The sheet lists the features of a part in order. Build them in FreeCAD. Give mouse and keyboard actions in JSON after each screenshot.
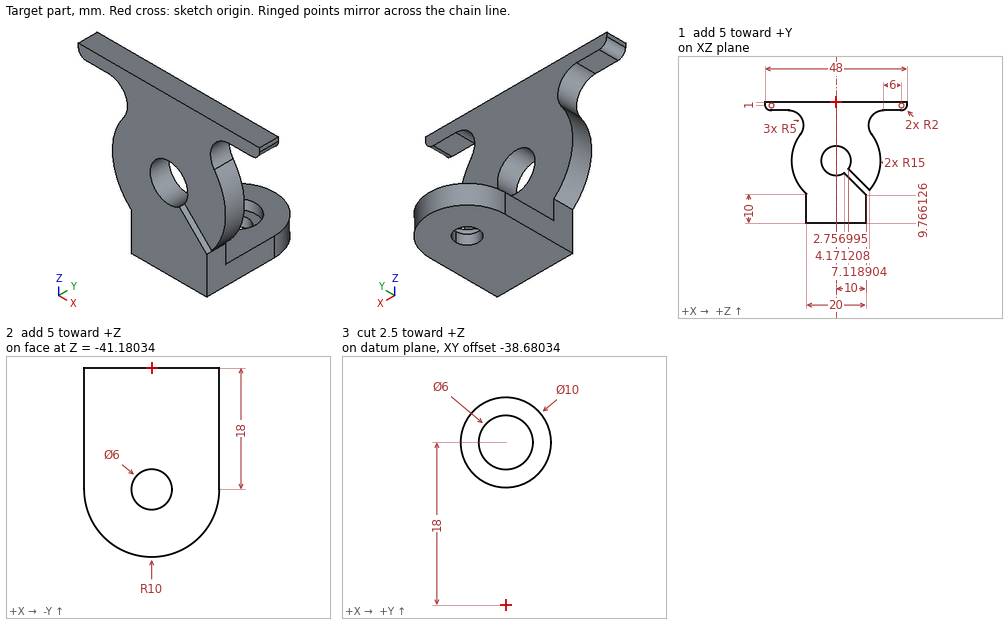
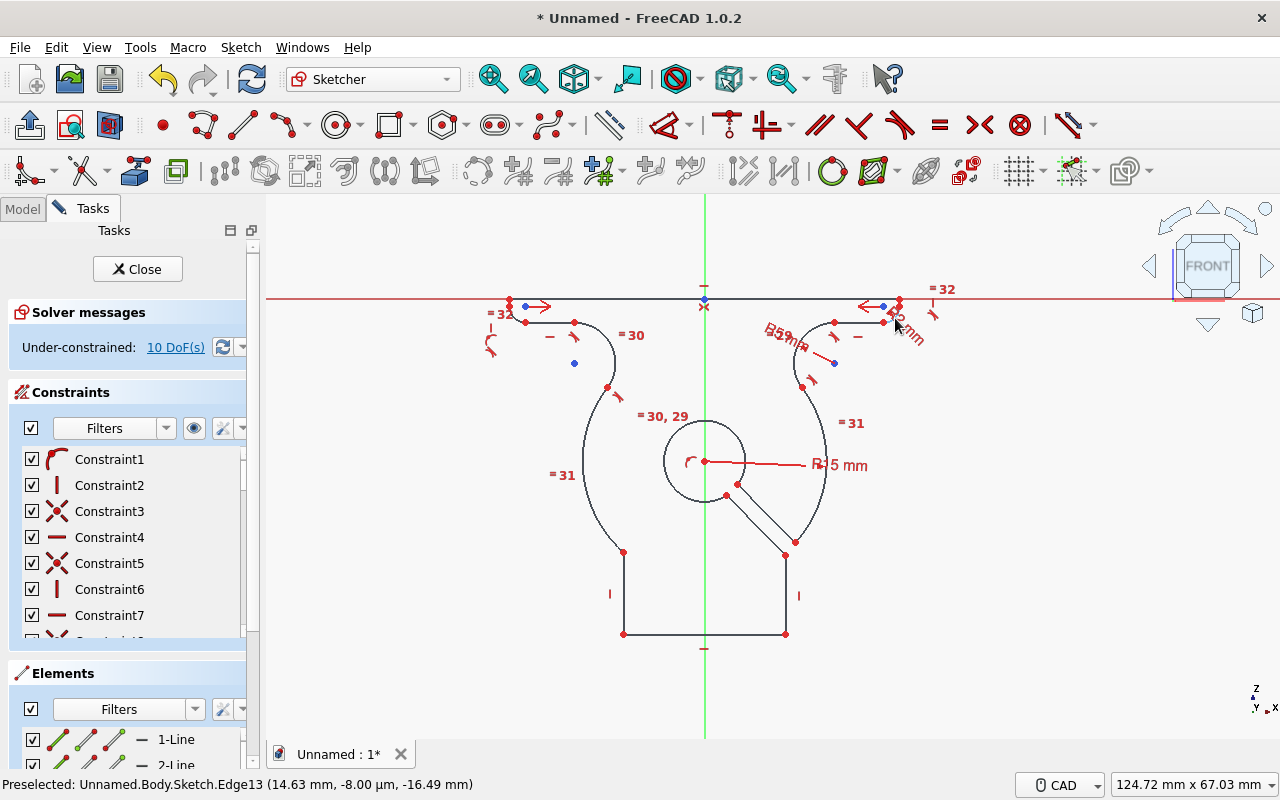
{"action": "scroll", "coordinate": [510, 303], "scroll_direction": "up", "scroll_amount": 8}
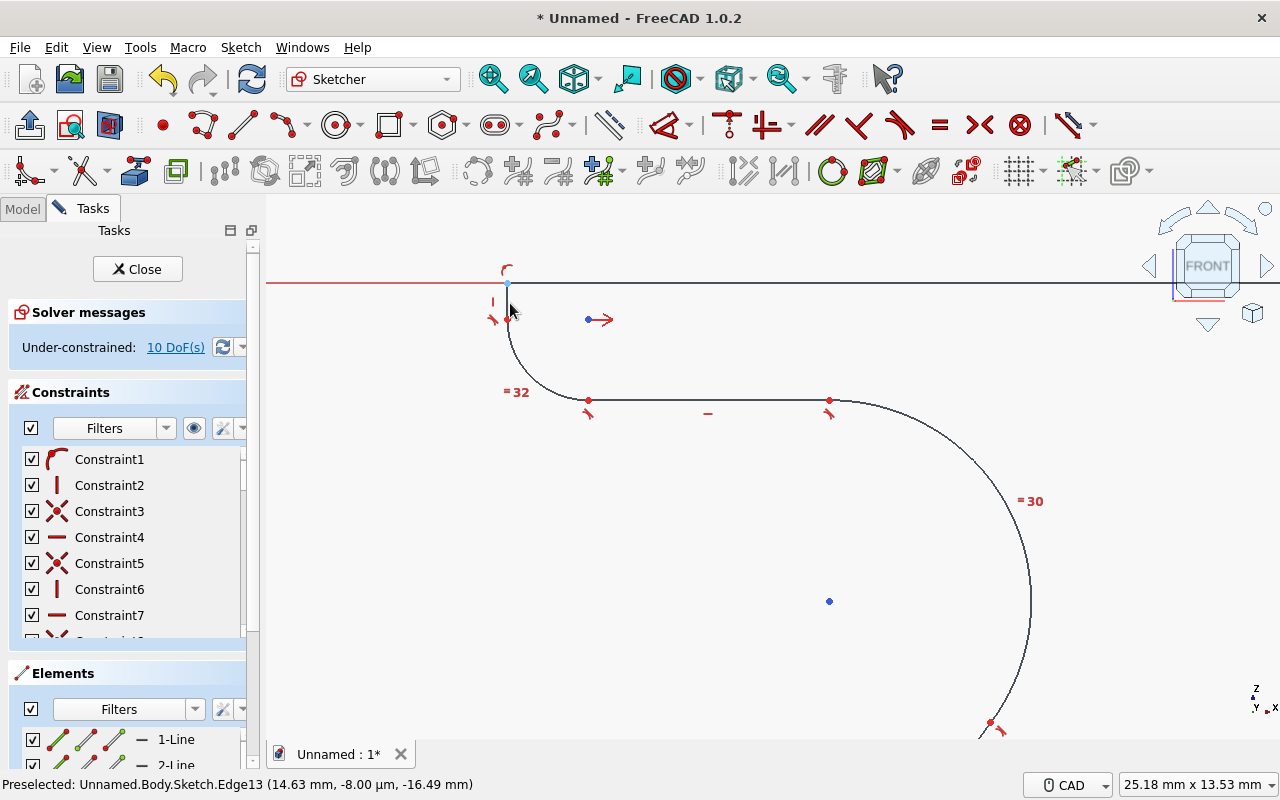
{"action": "left_click", "coordinate": [507, 301]}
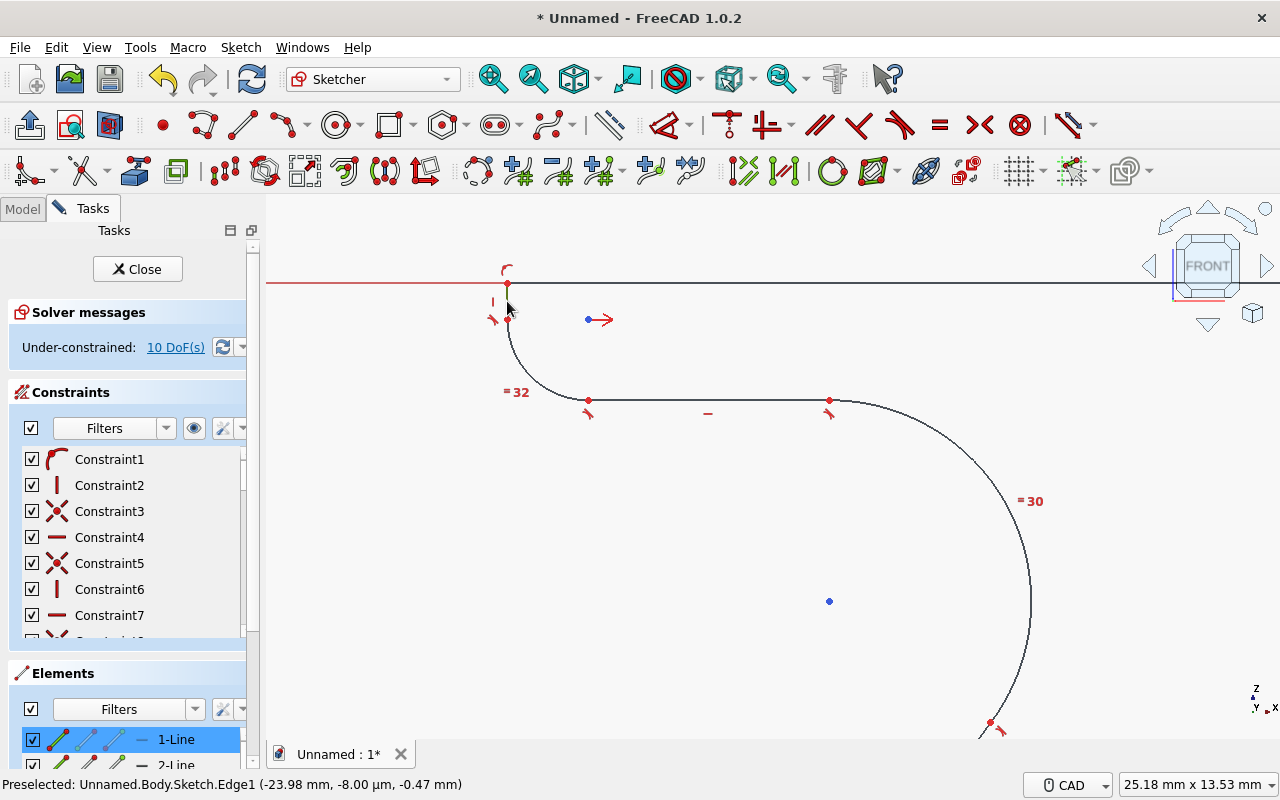
{"action": "left_click", "coordinate": [692, 126]}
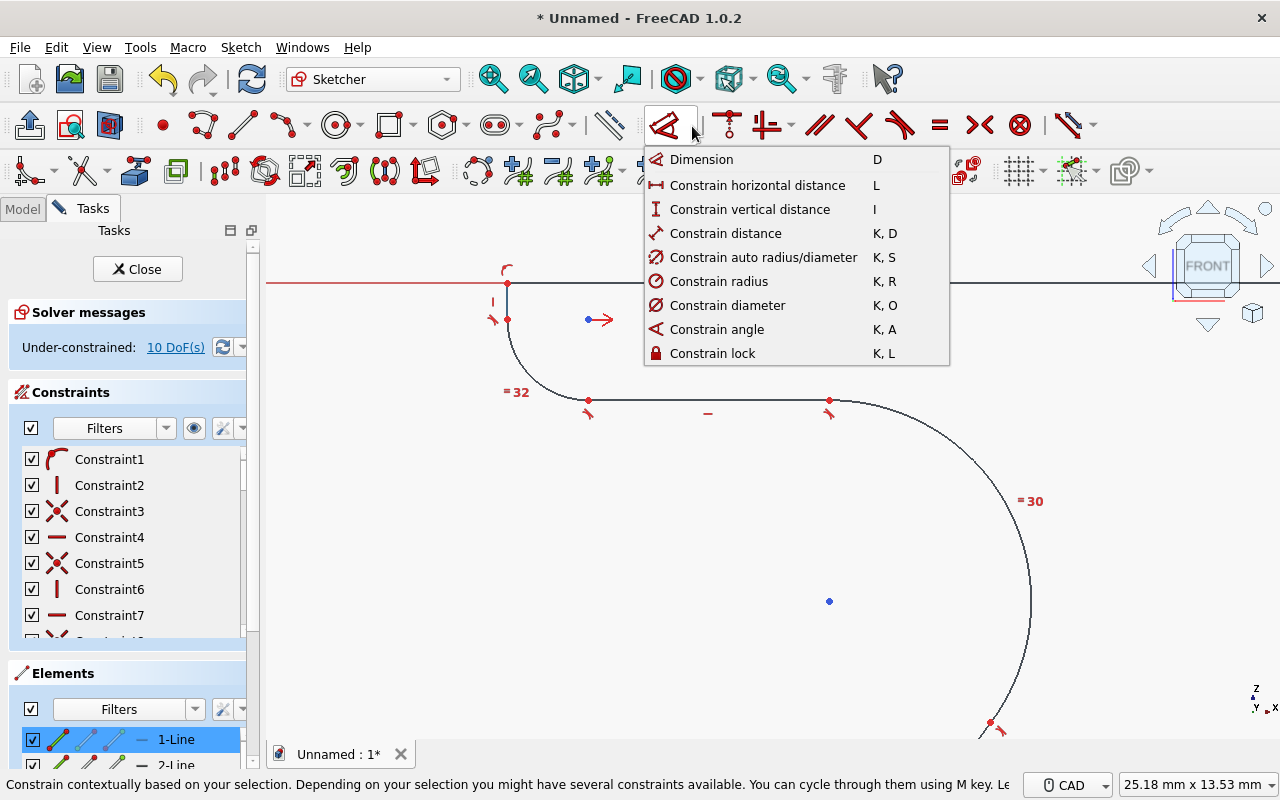
{"action": "left_click", "coordinate": [797, 209]}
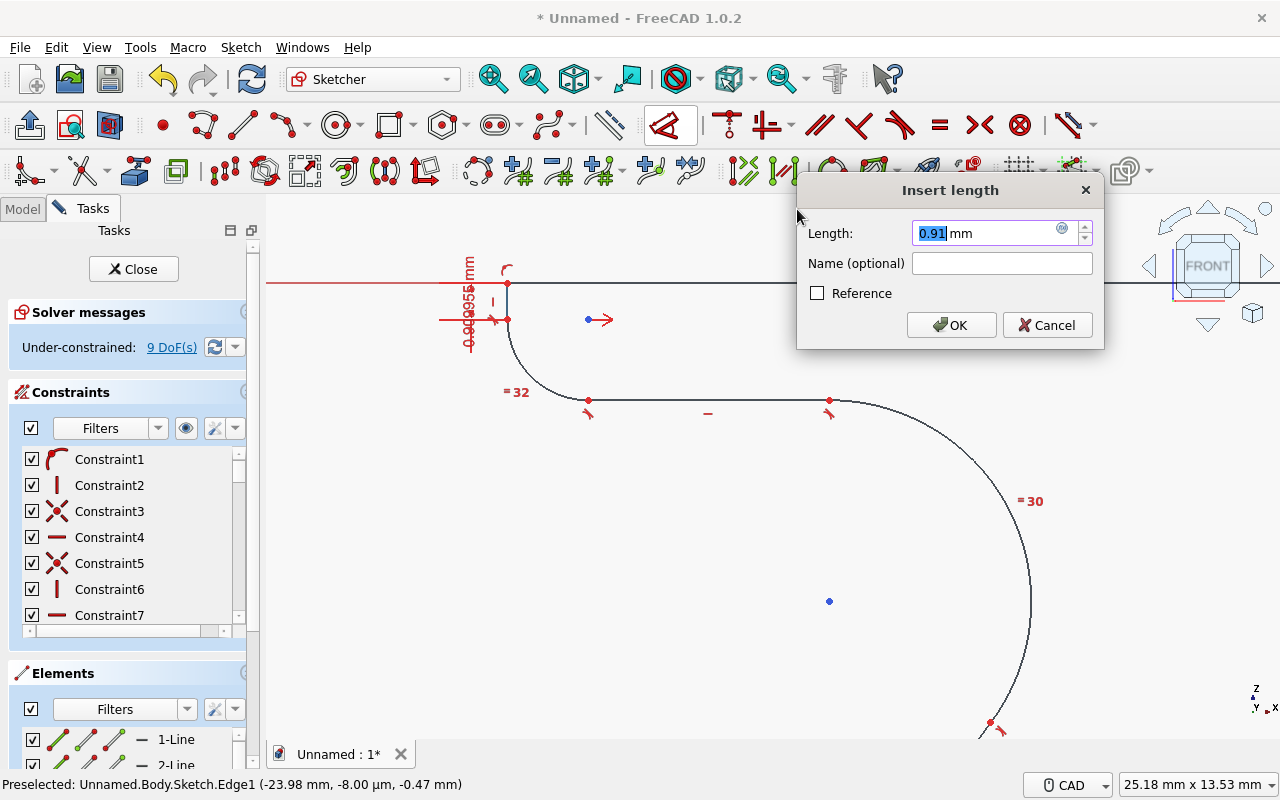
{"action": "type", "text": "1"}
{"action": "key", "text": "Return"}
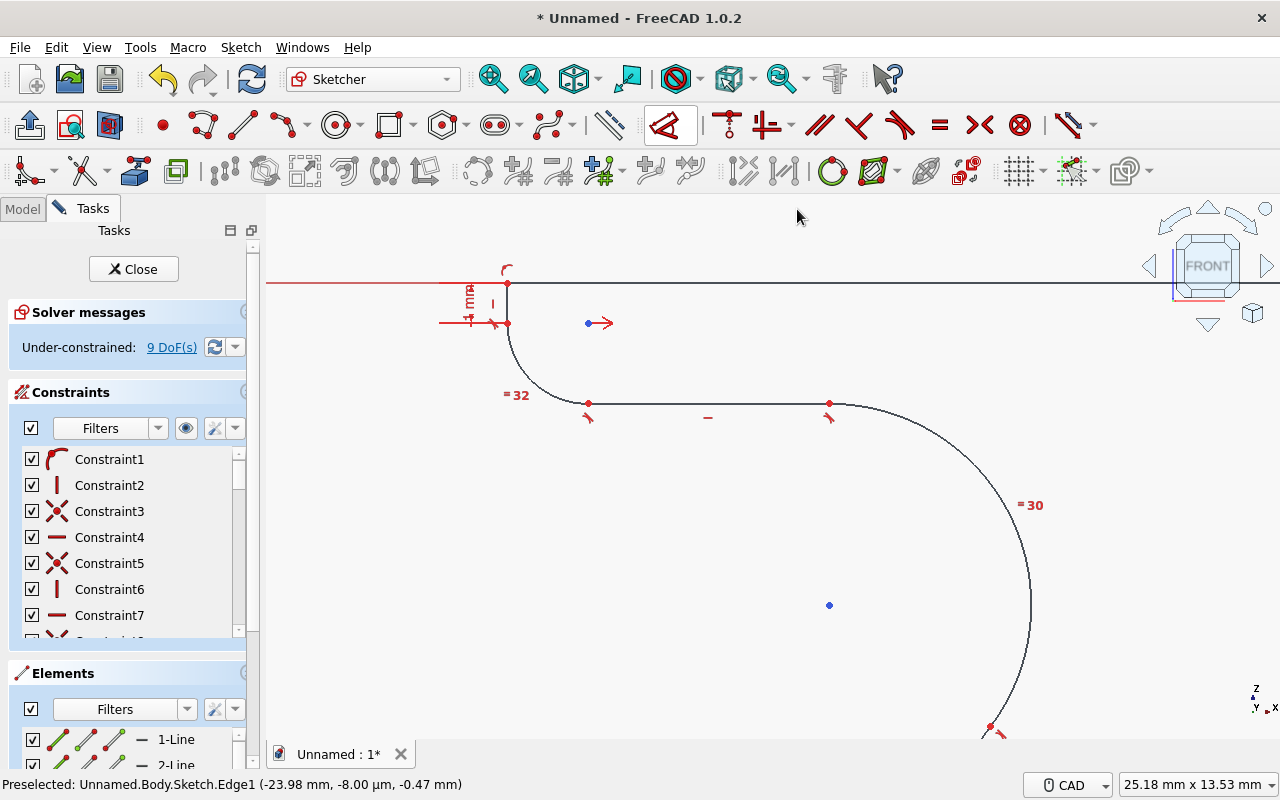
{"action": "scroll", "coordinate": [510, 303], "scroll_direction": "down", "scroll_amount": 8}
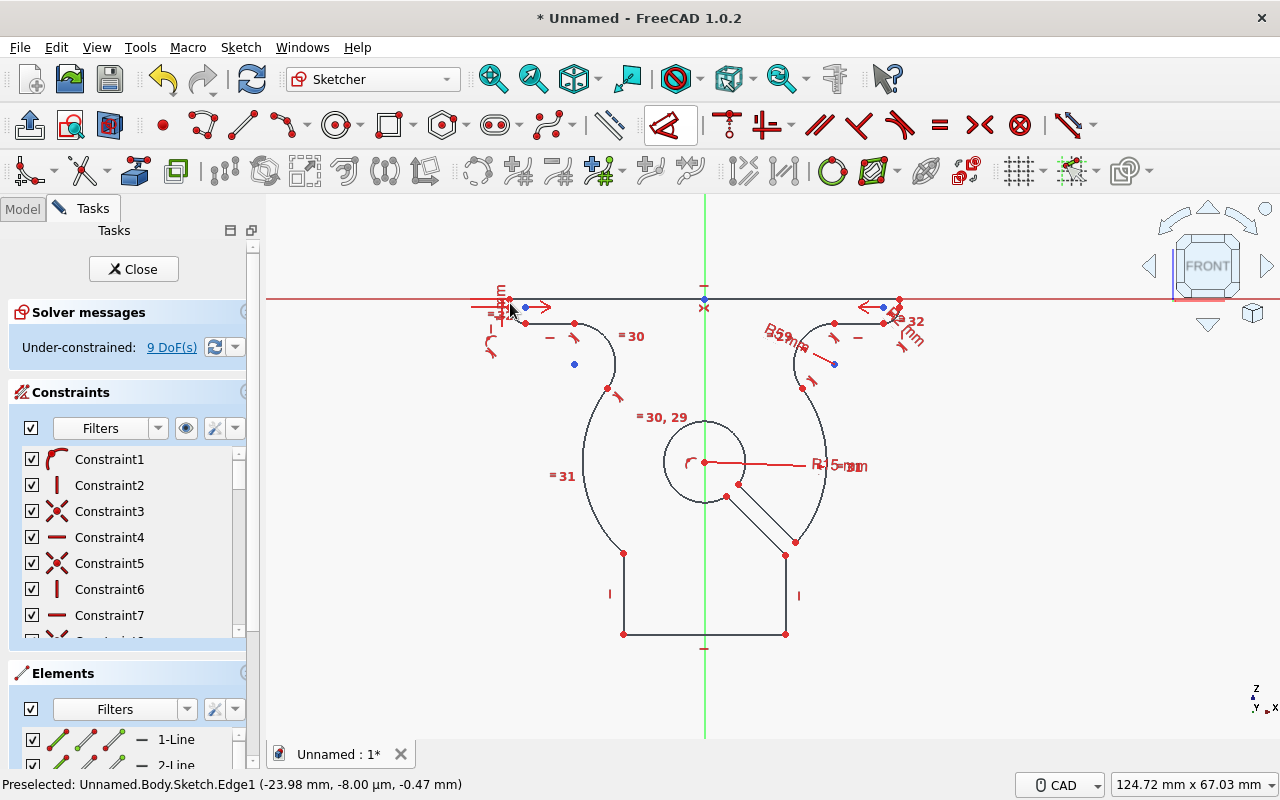
{"action": "left_click", "coordinate": [869, 324]}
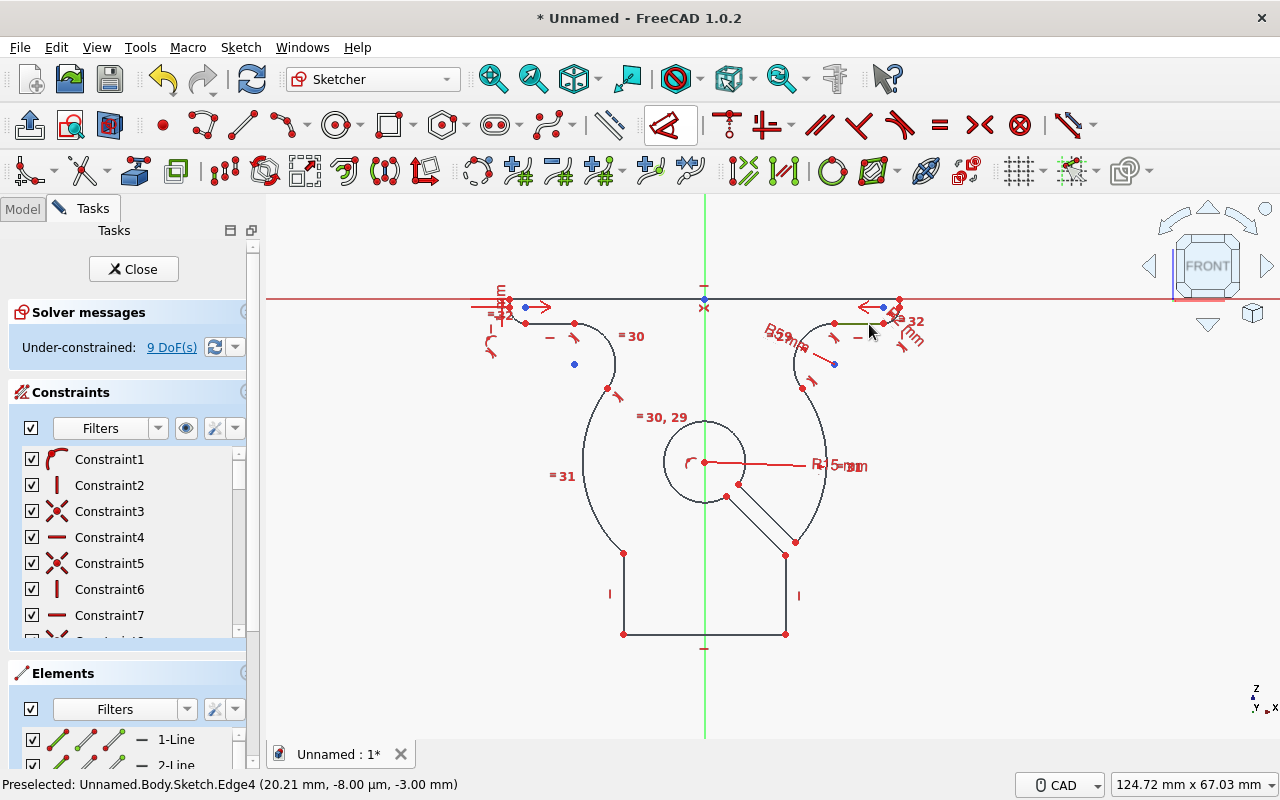
{"action": "key", "text": "l"}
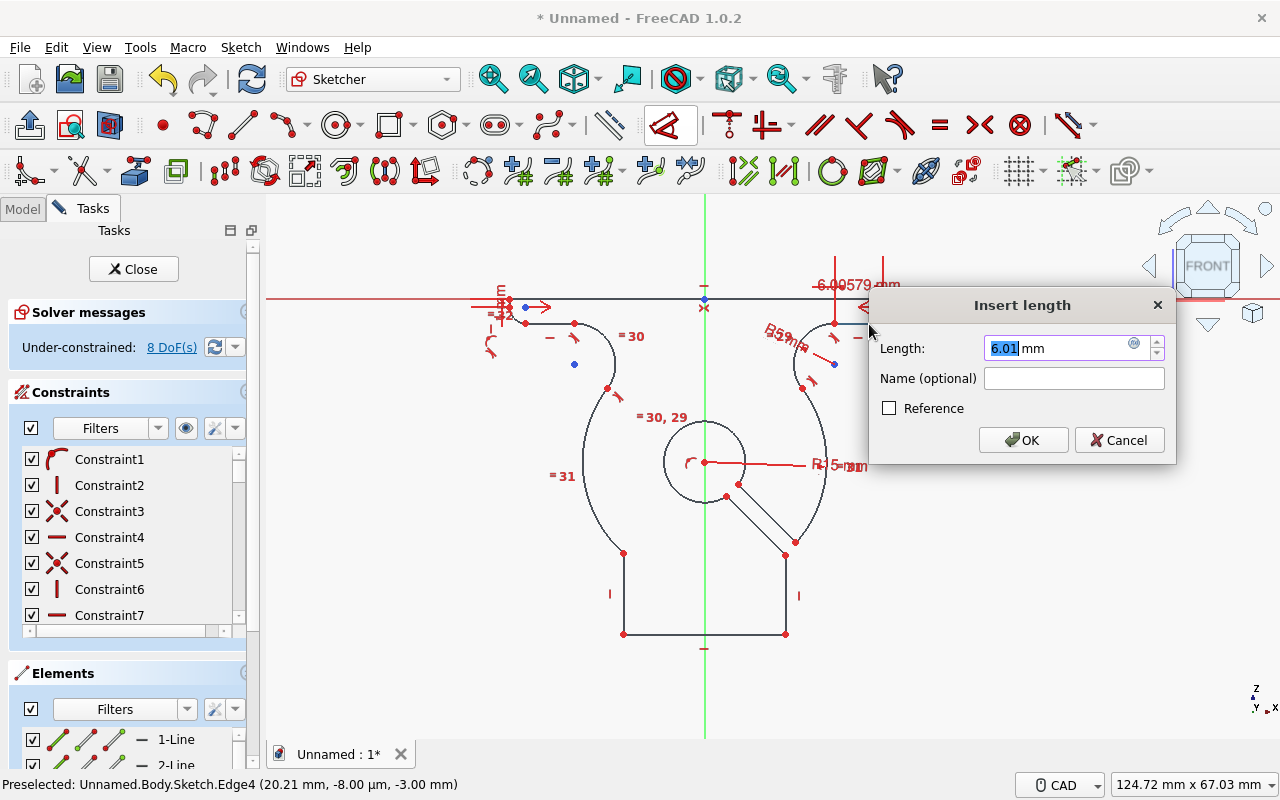
{"action": "type", "text": "6"}
{"action": "key", "text": "Return"}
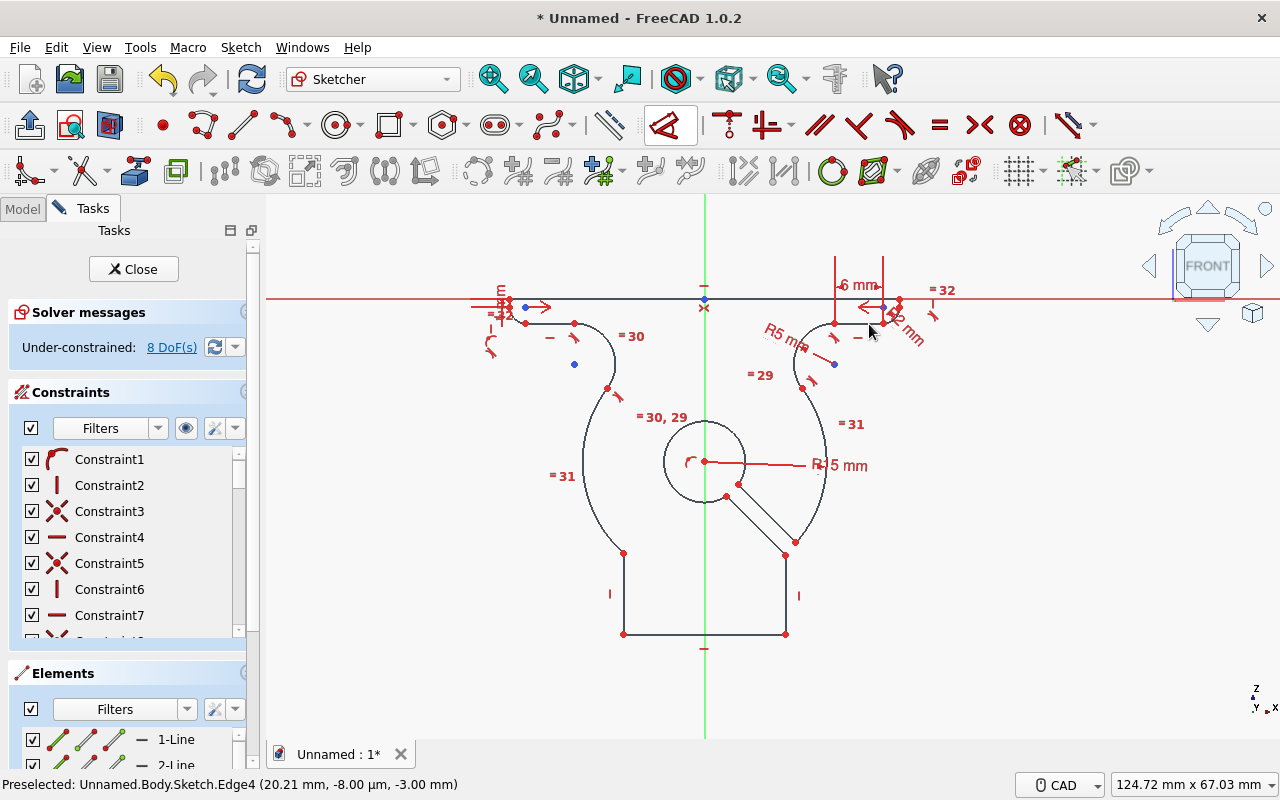
{"action": "left_click", "coordinate": [627, 299]}